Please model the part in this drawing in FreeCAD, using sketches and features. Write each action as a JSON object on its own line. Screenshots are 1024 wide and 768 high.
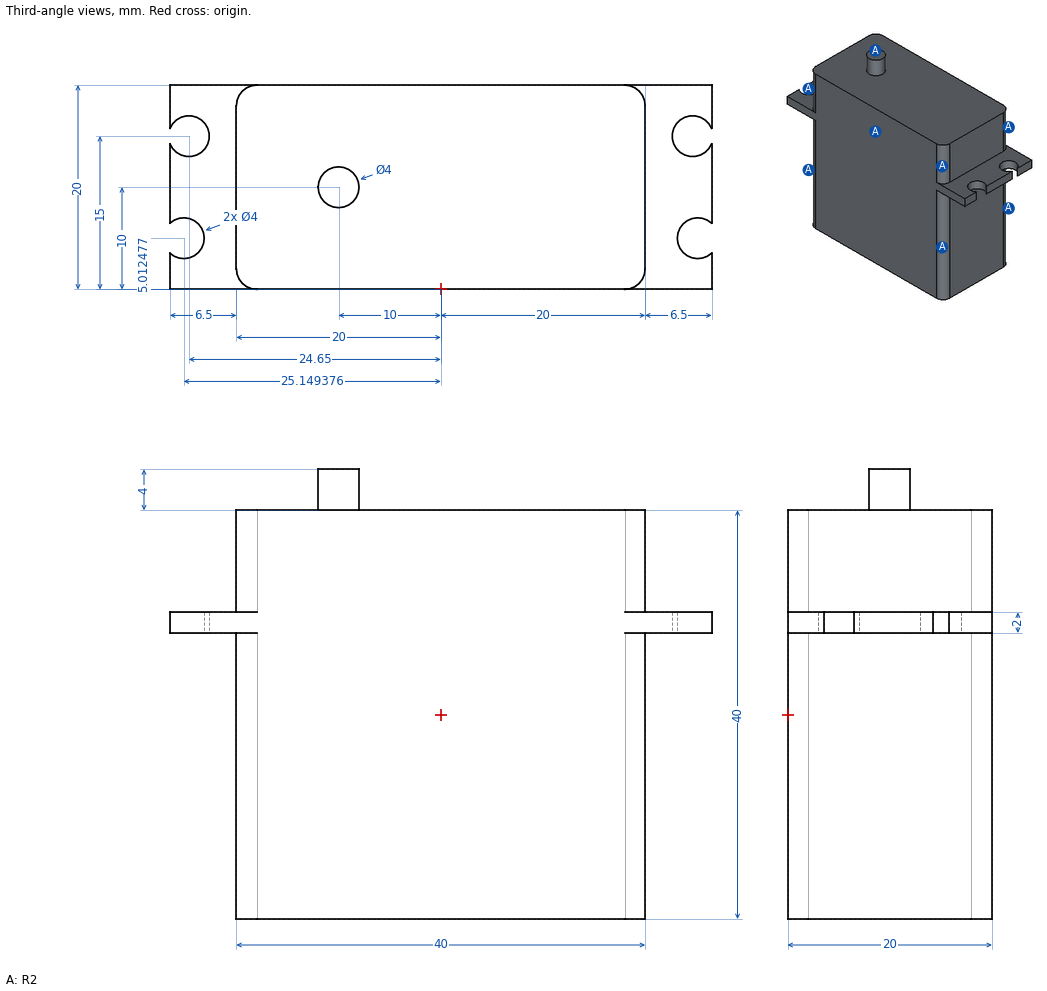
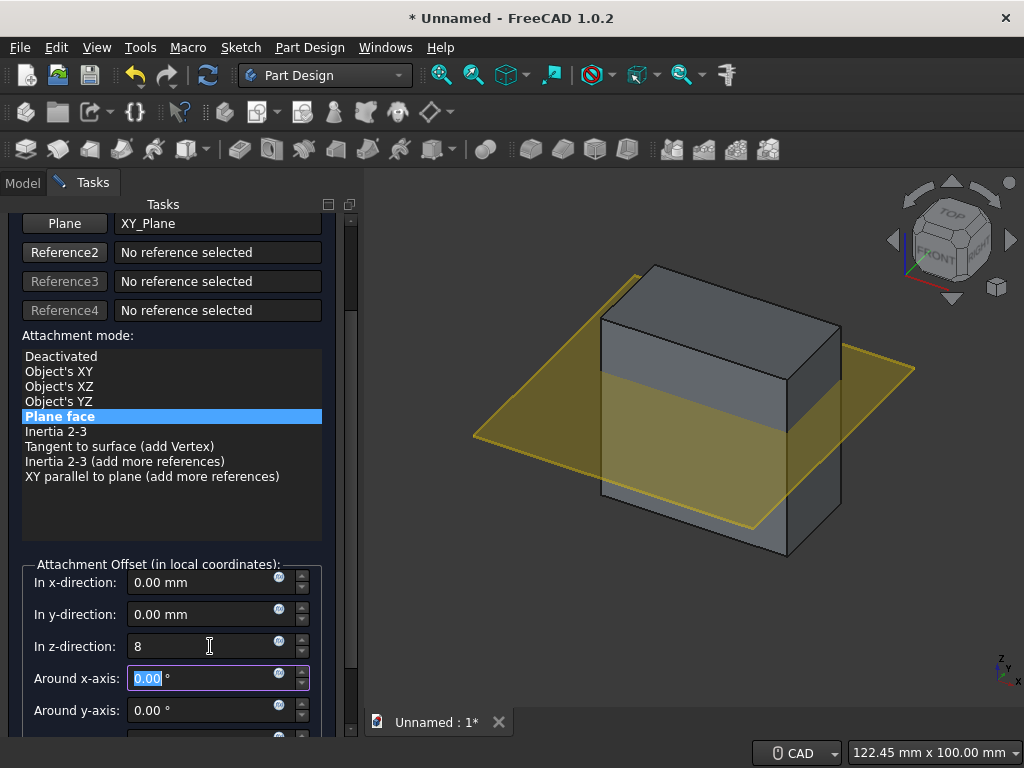
{"action": "scroll", "coordinate": [351, 475], "scroll_direction": "up", "scroll_amount": 3}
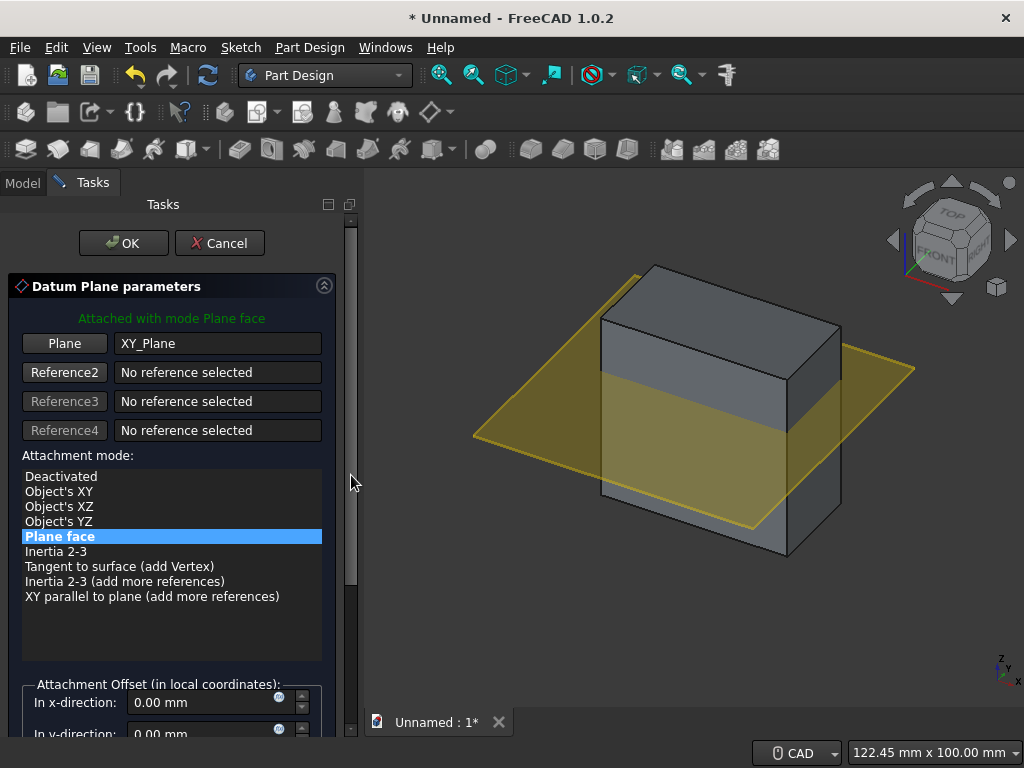
{"action": "left_click", "coordinate": [124, 243]}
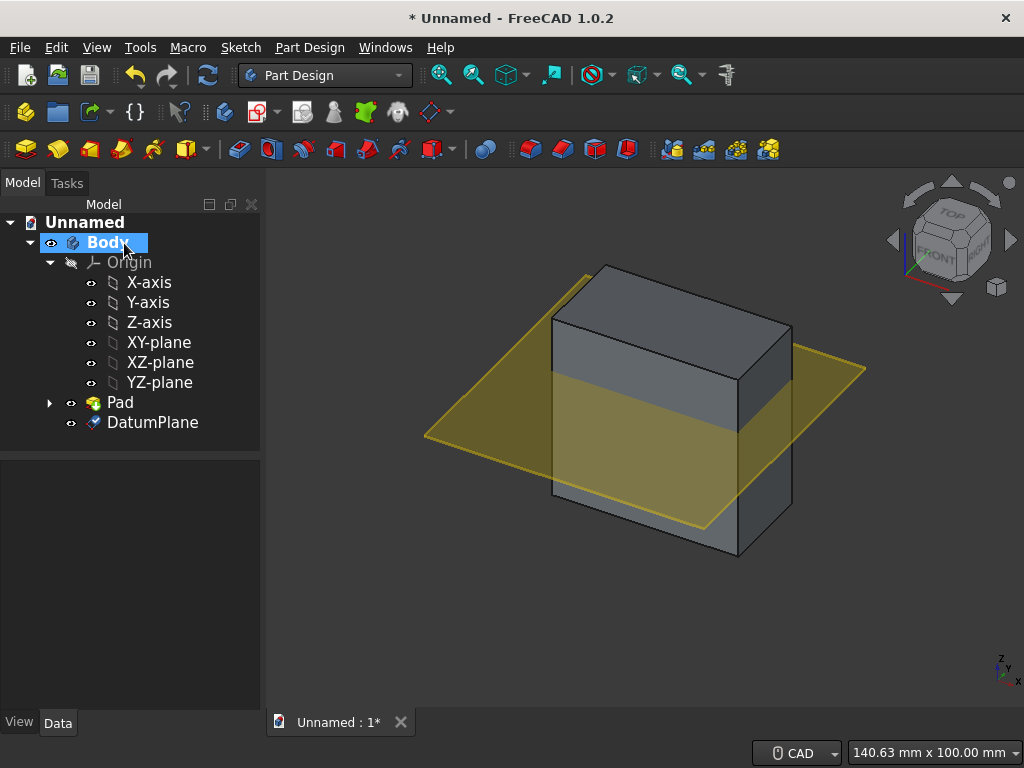
{"action": "left_click", "coordinate": [116, 423]}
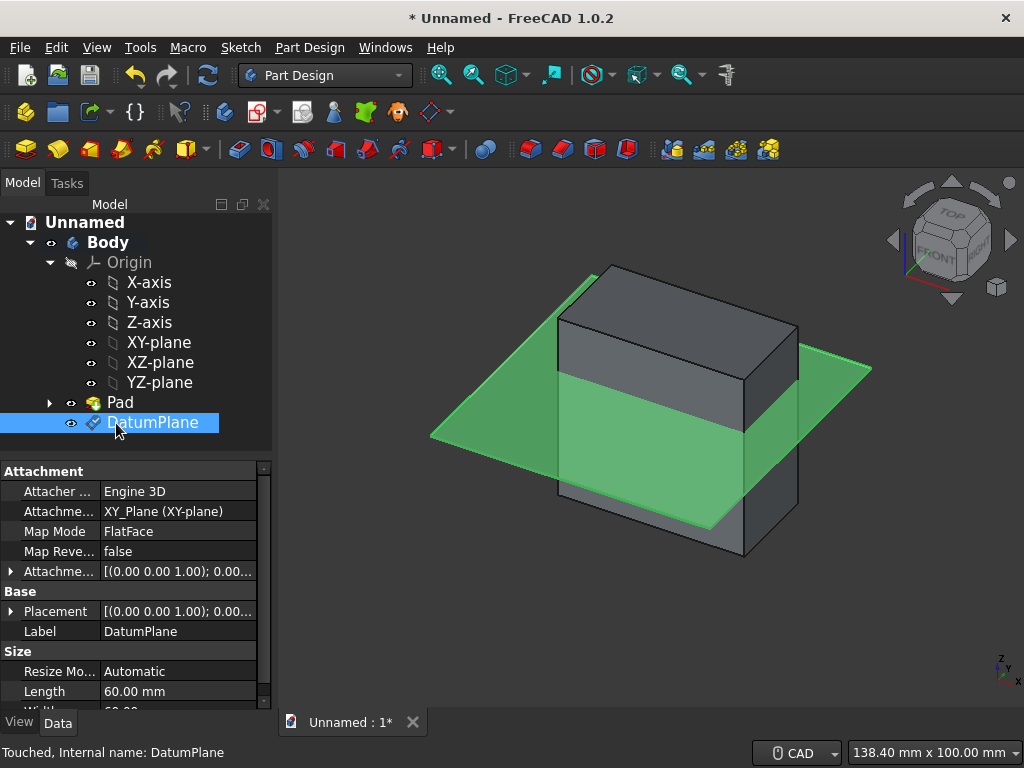
{"action": "left_click", "coordinate": [258, 112]}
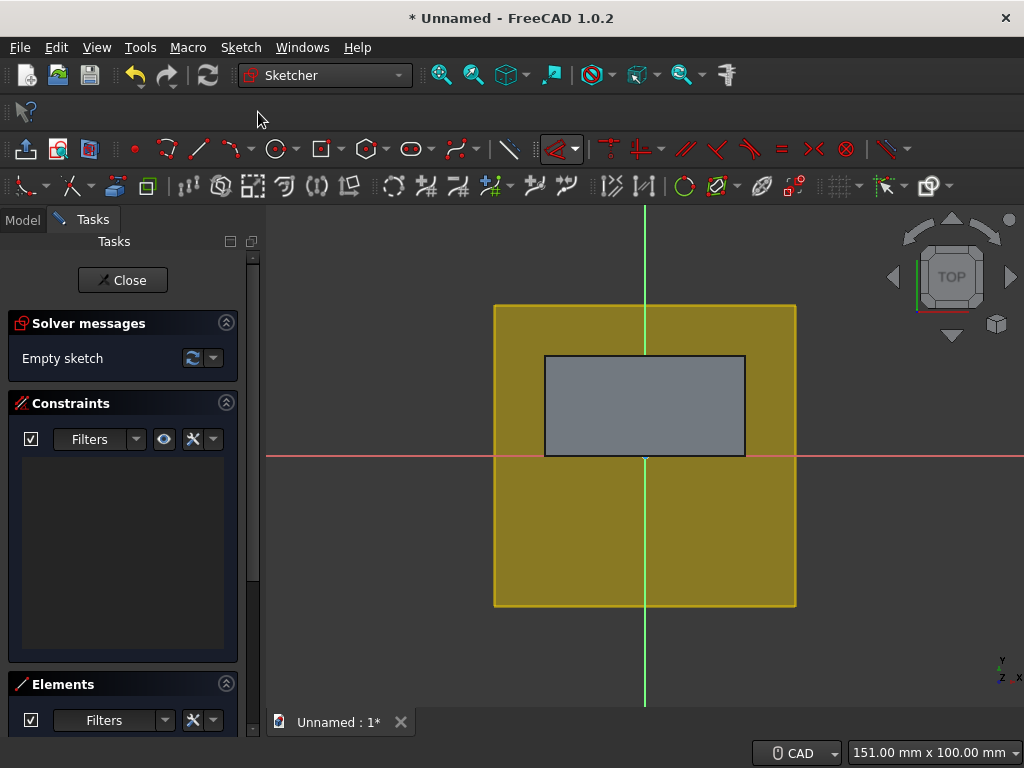
{"action": "left_click", "coordinate": [90, 150]}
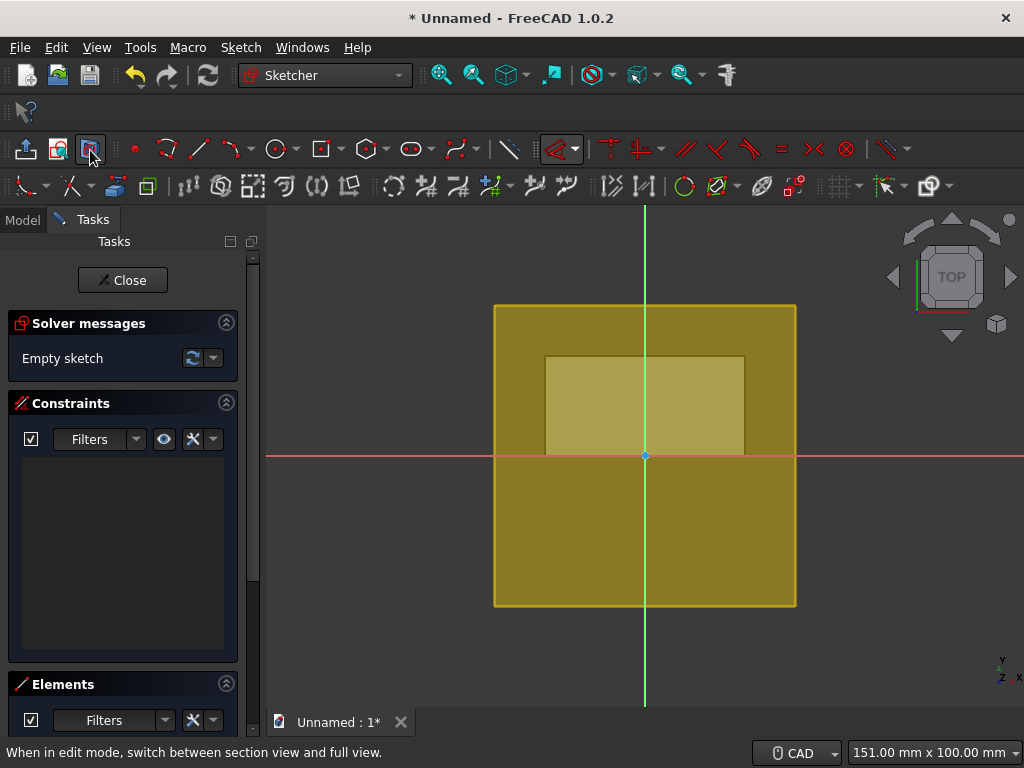
{"action": "scroll", "coordinate": [784, 304], "scroll_direction": "up", "scroll_amount": 2}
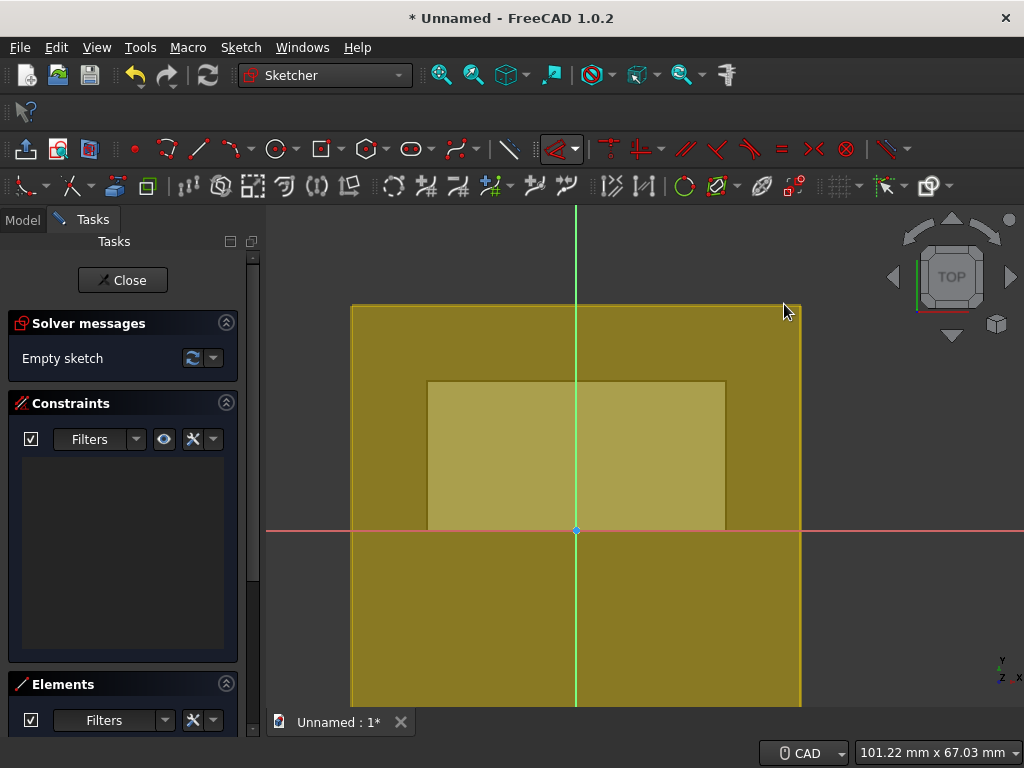
{"action": "key", "text": "g r"}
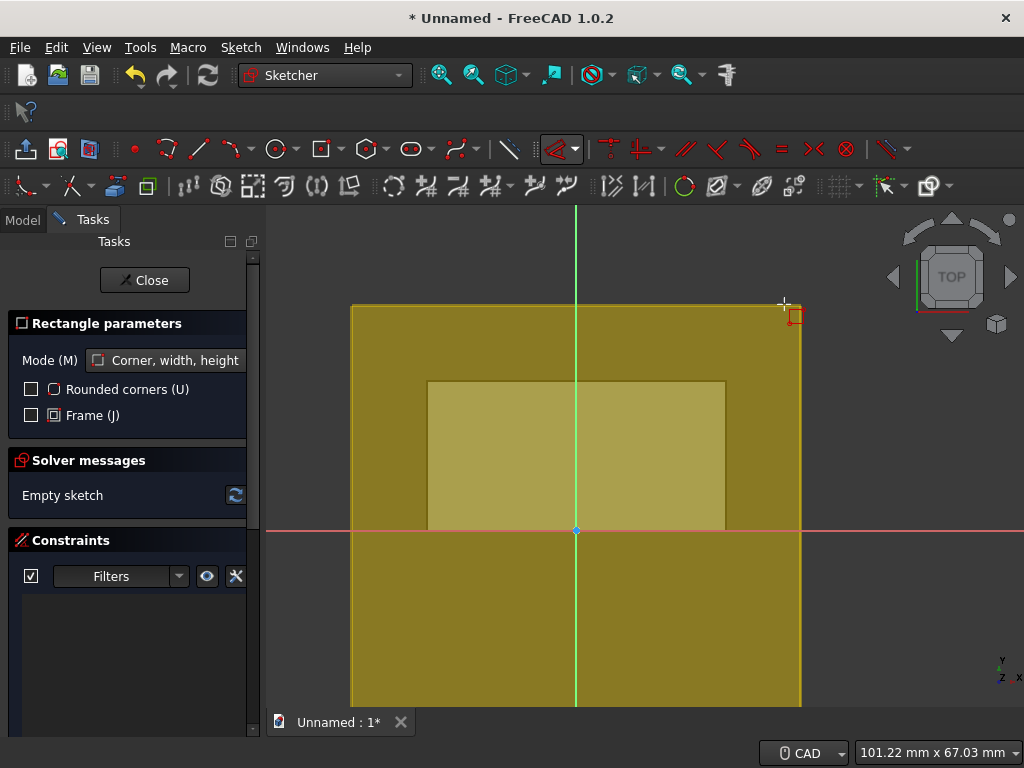
{"action": "left_click", "coordinate": [378, 381]}
{"action": "left_click", "coordinate": [427, 531]}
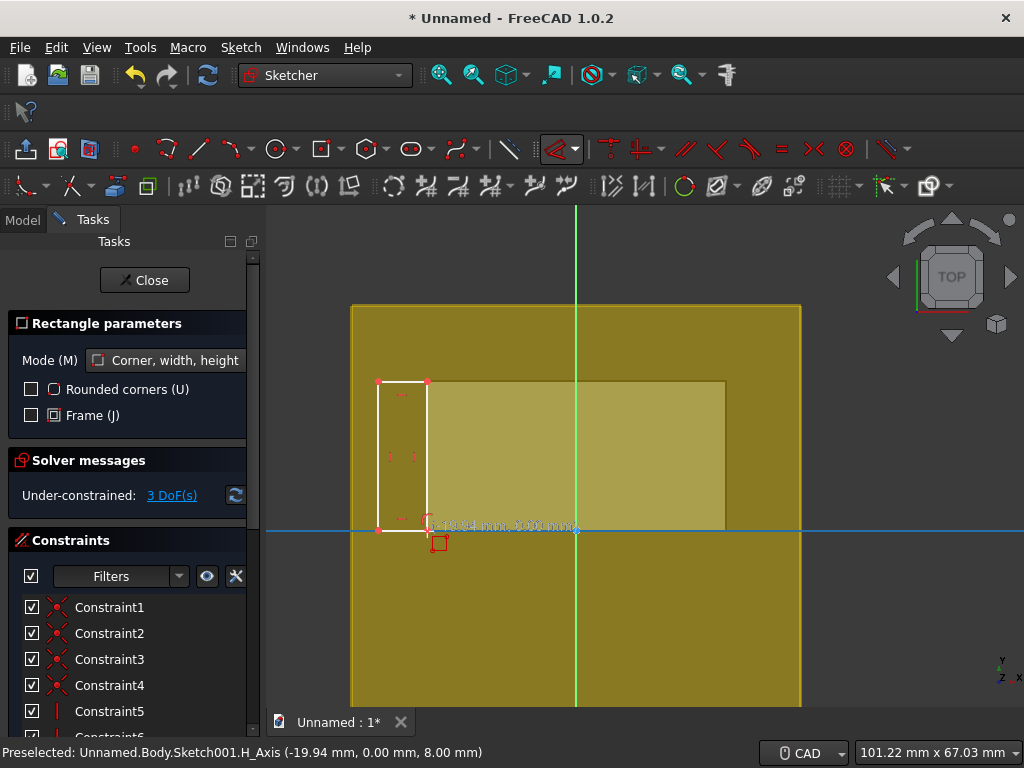
{"action": "left_click", "coordinate": [726, 381]}
{"action": "left_click", "coordinate": [775, 531]}
{"action": "key", "text": "Escape"}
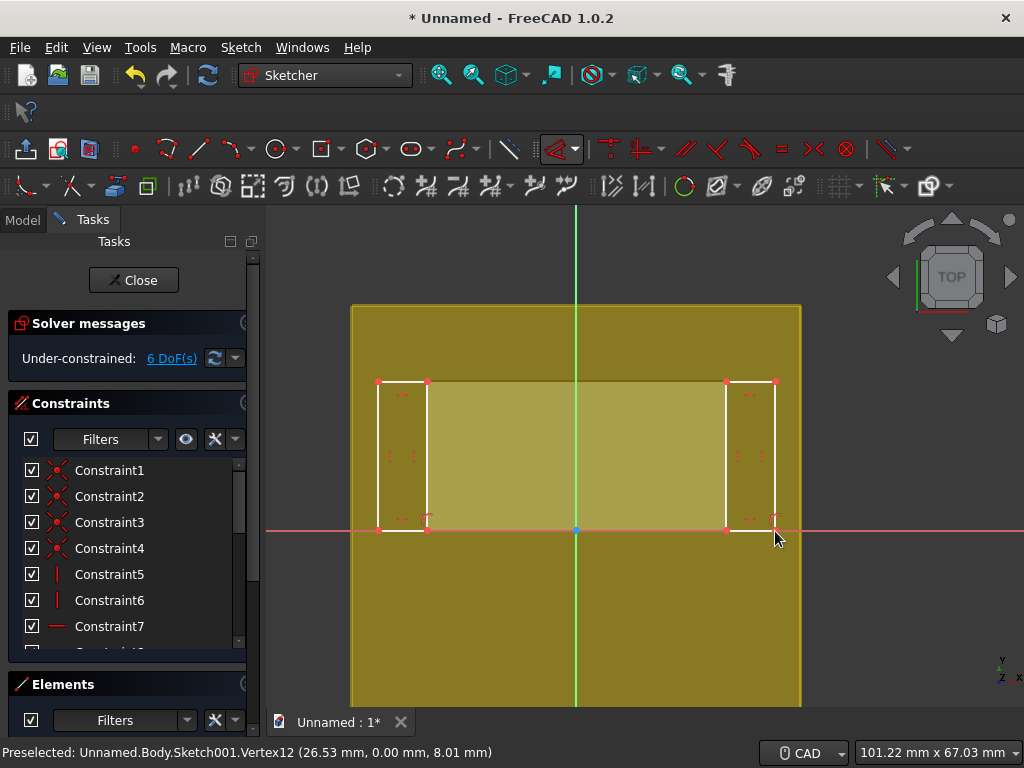
{"action": "left_click", "coordinate": [378, 427]}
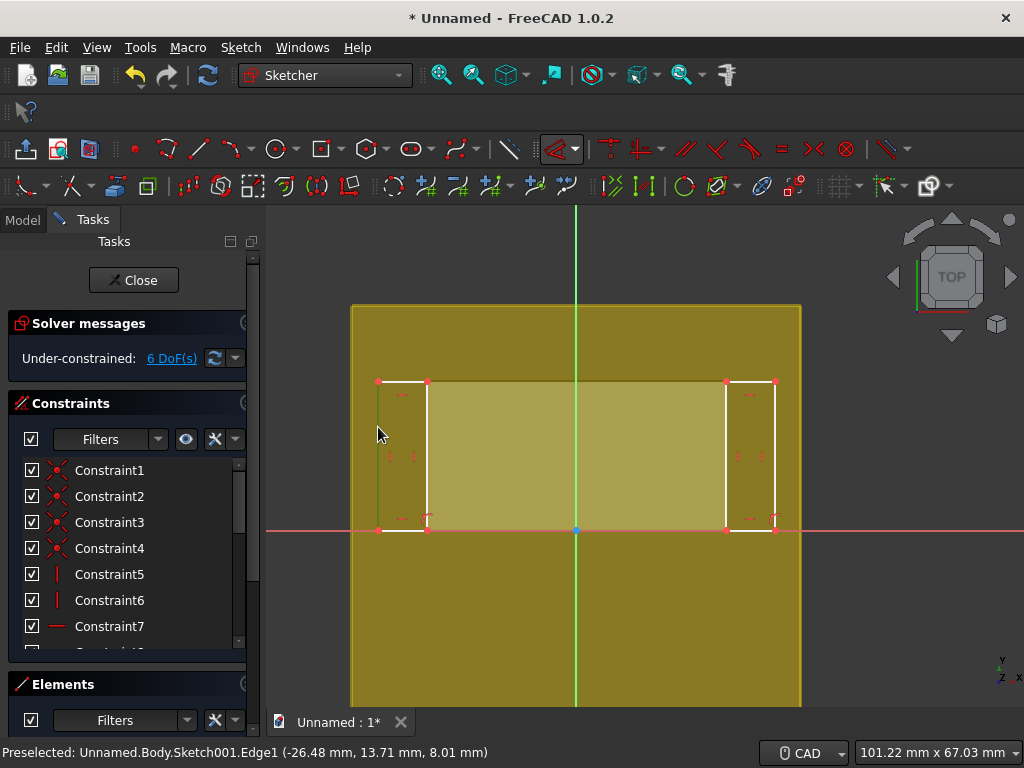
{"action": "left_click", "coordinate": [578, 150]}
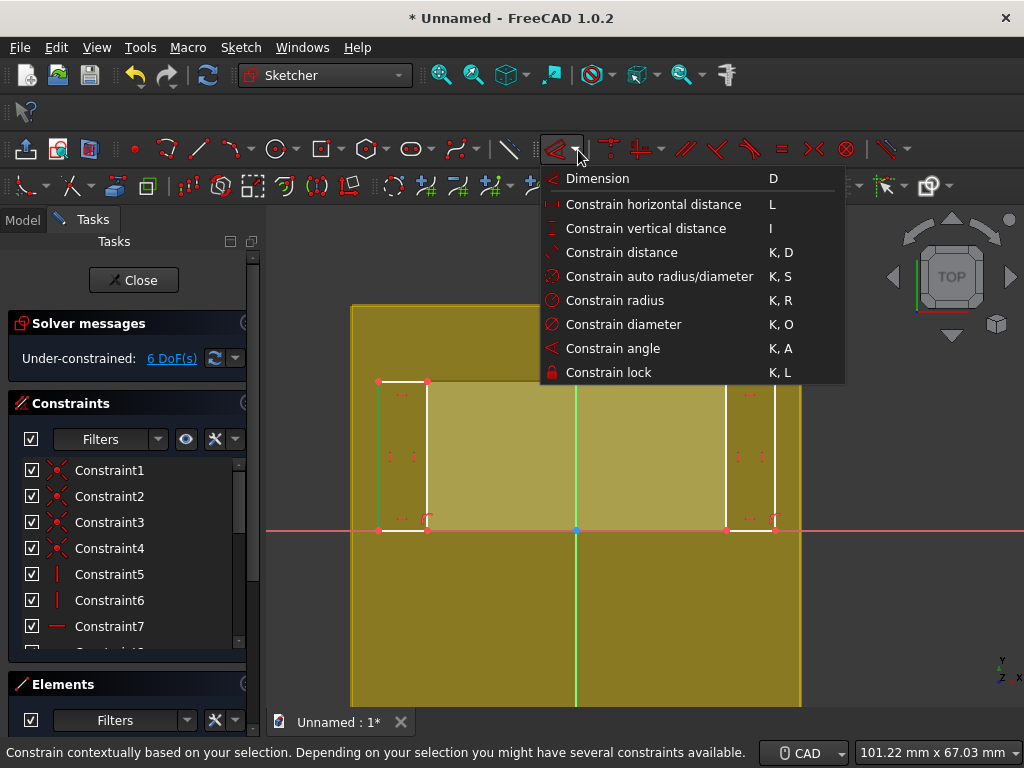
{"action": "left_click", "coordinate": [693, 228]}